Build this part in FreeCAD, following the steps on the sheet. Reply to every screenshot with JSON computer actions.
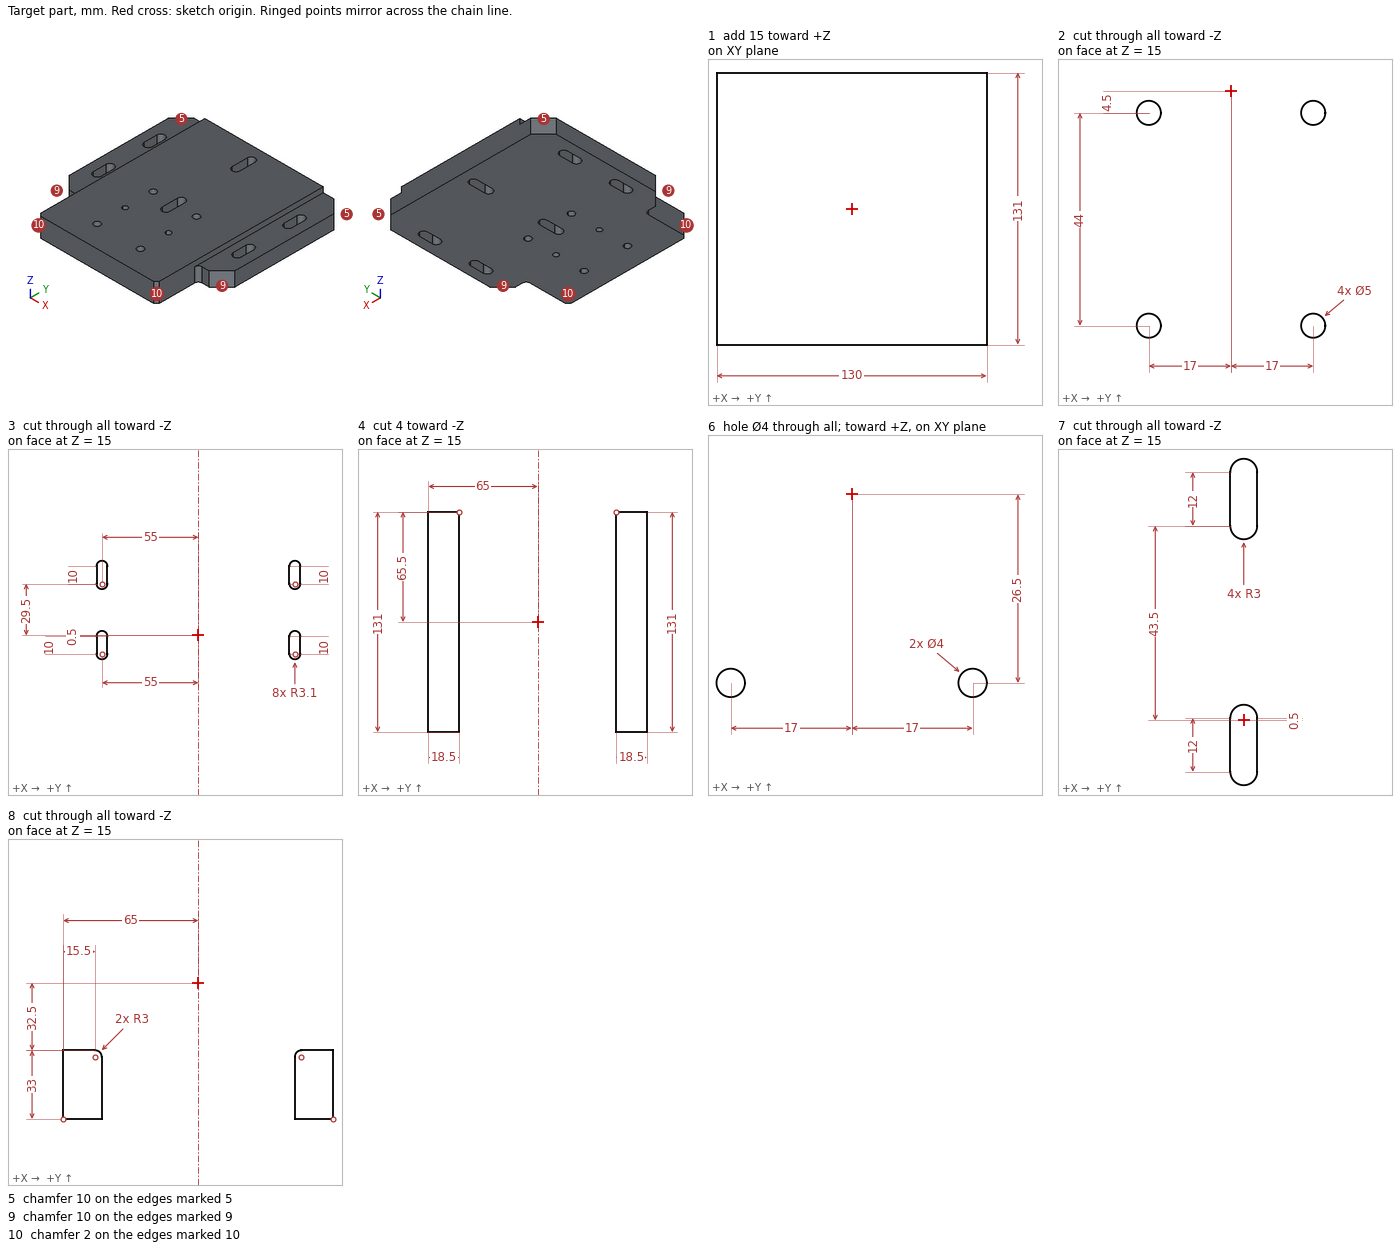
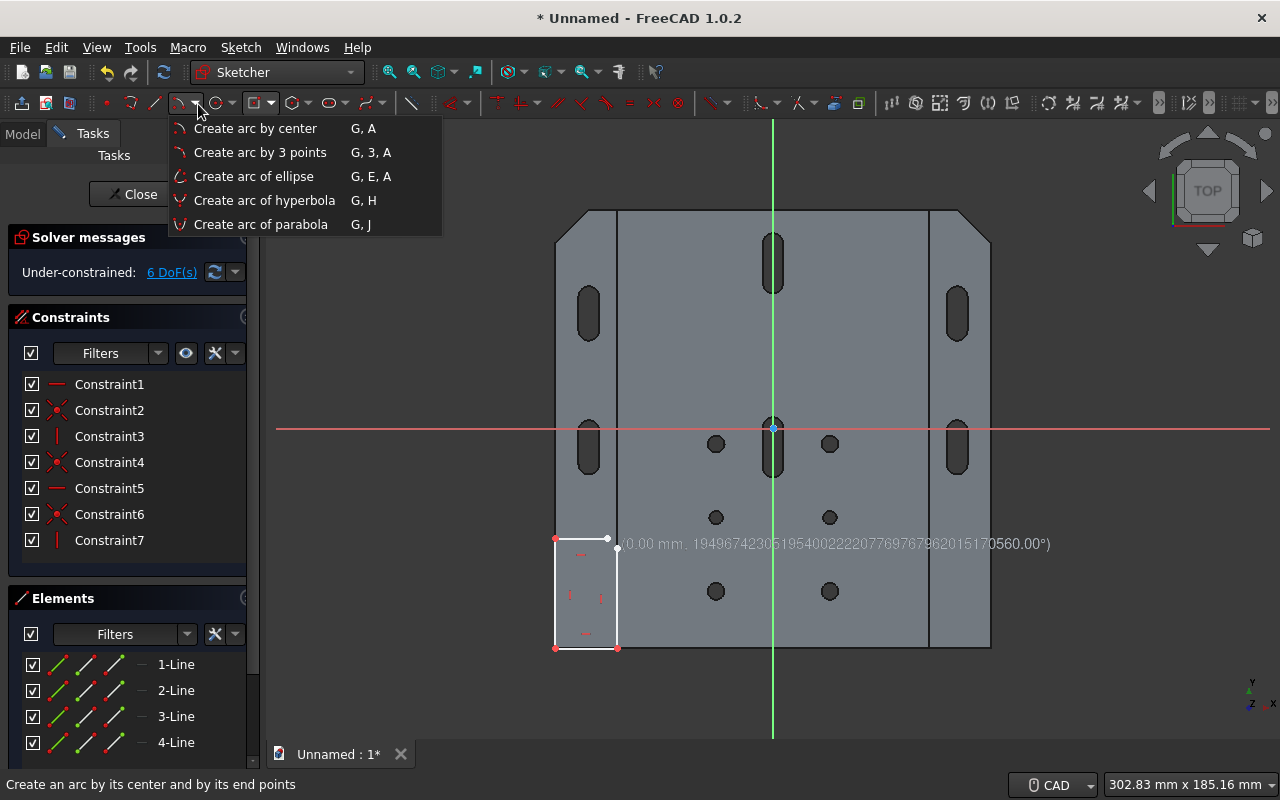
{"action": "left_click", "coordinate": [306, 152]}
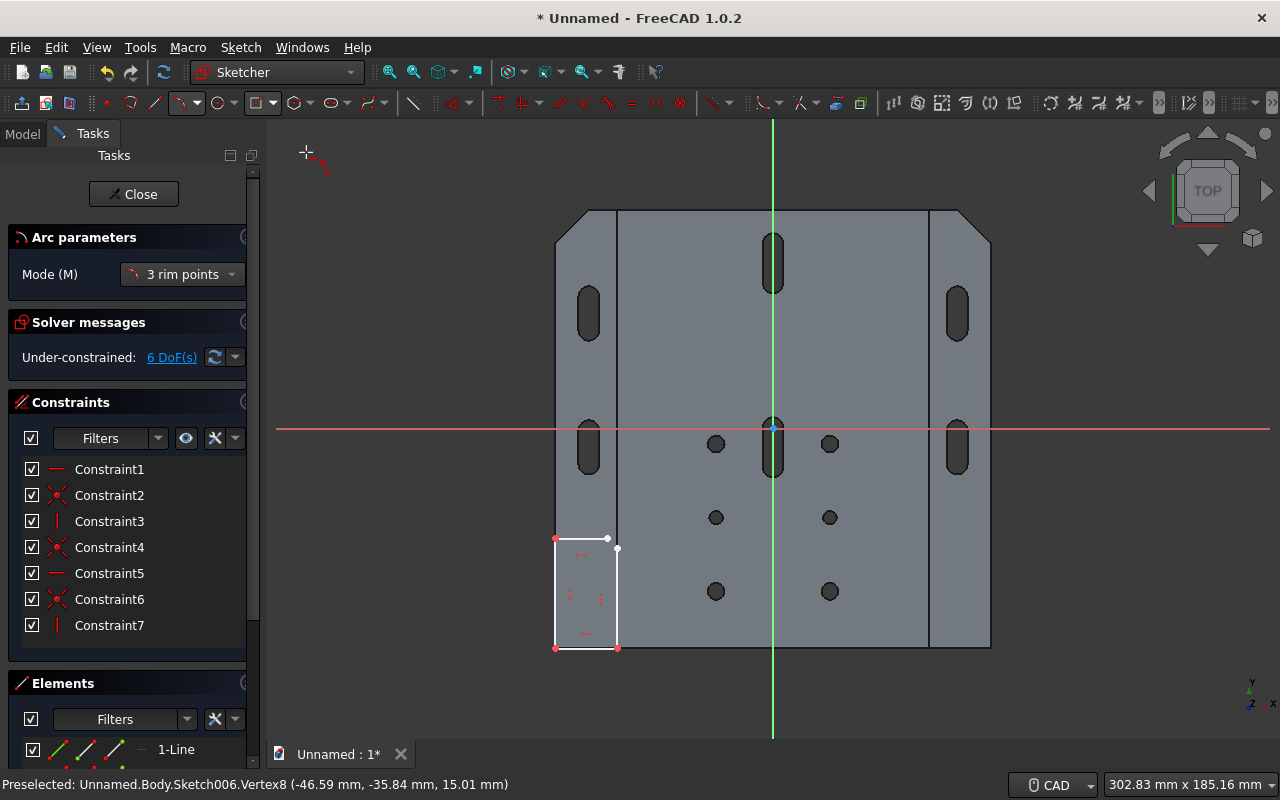
{"action": "left_click", "coordinate": [617, 549]}
{"action": "left_click", "coordinate": [607, 539]}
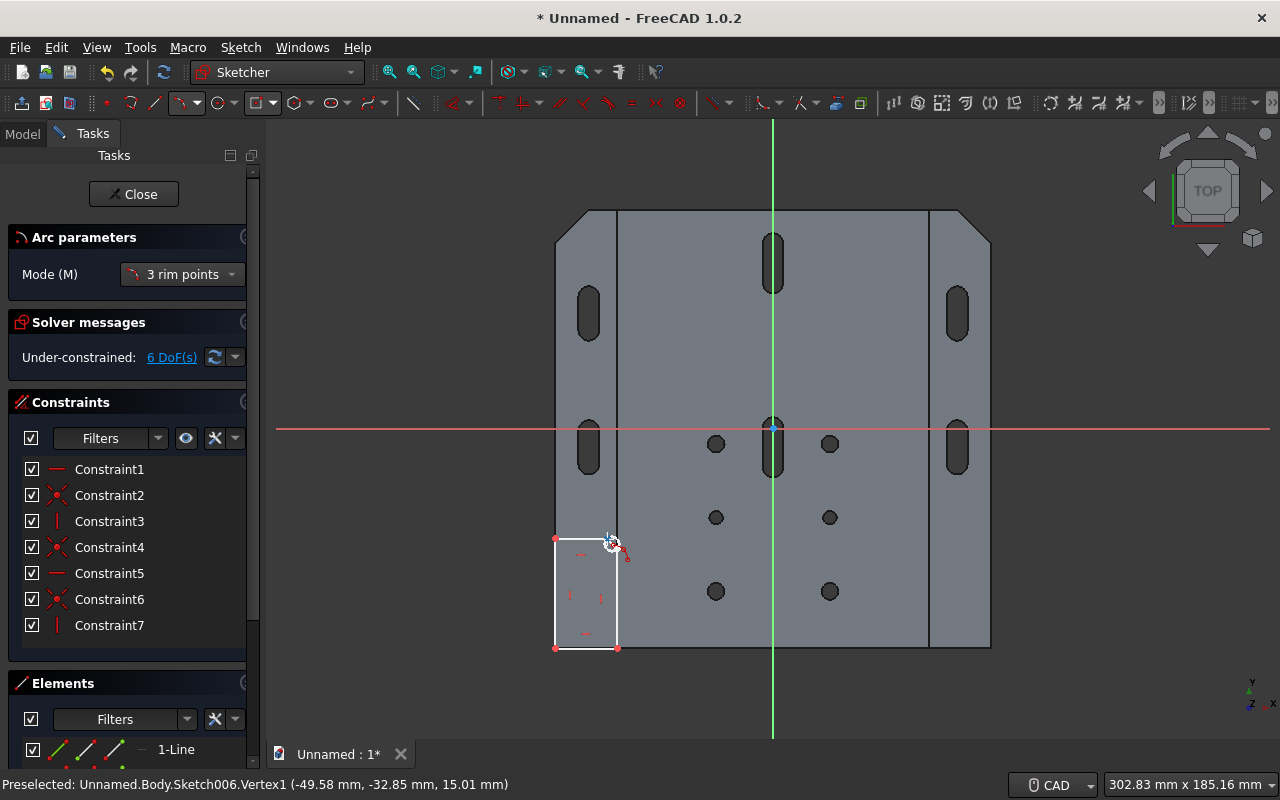
{"action": "scroll", "coordinate": [614, 541], "scroll_direction": "up", "scroll_amount": 9}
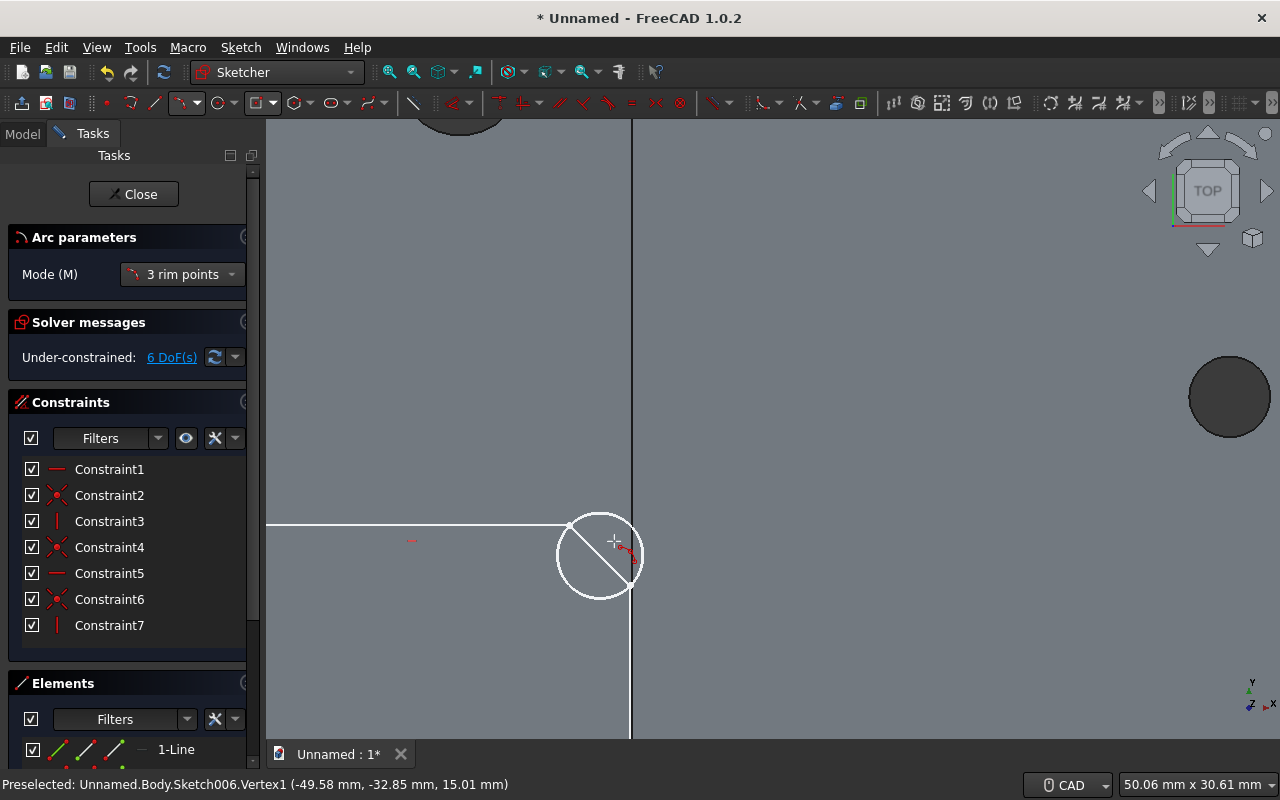
{"action": "left_click", "coordinate": [614, 536]}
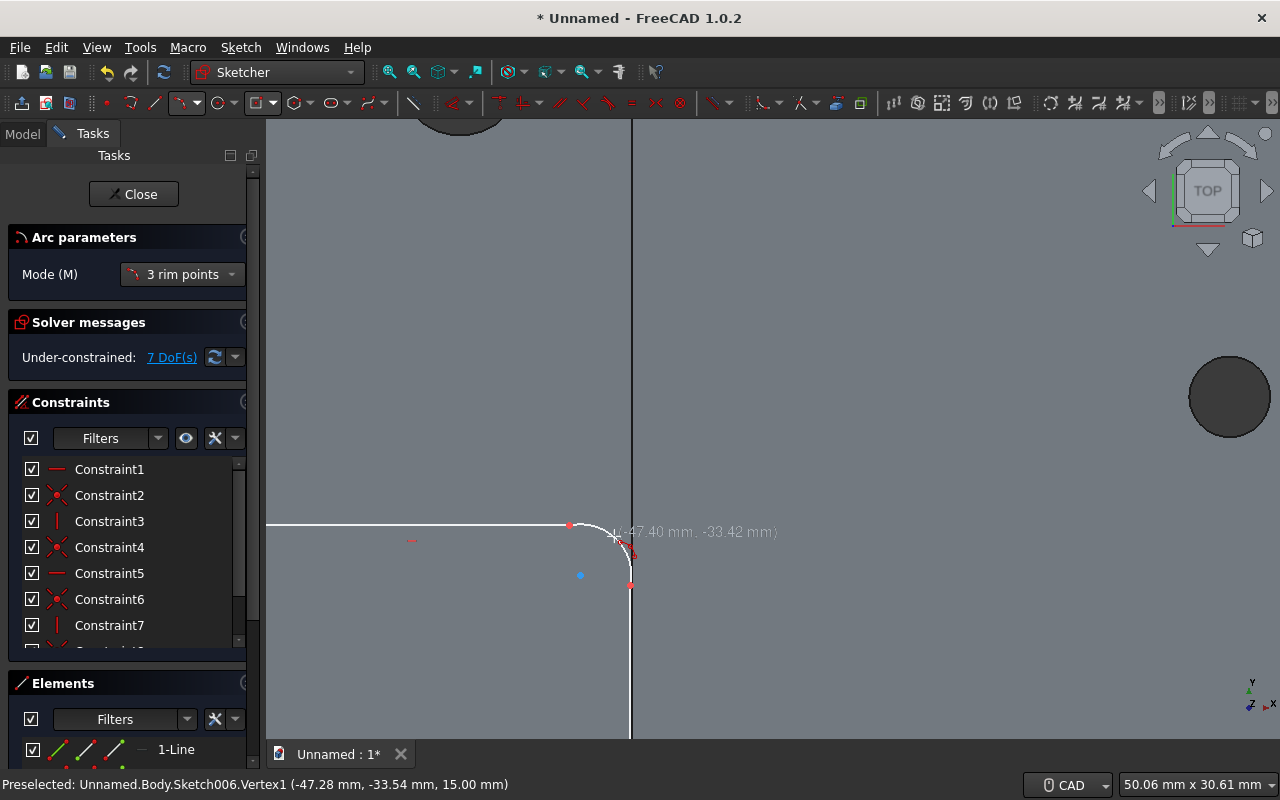
{"action": "key", "text": "g m"}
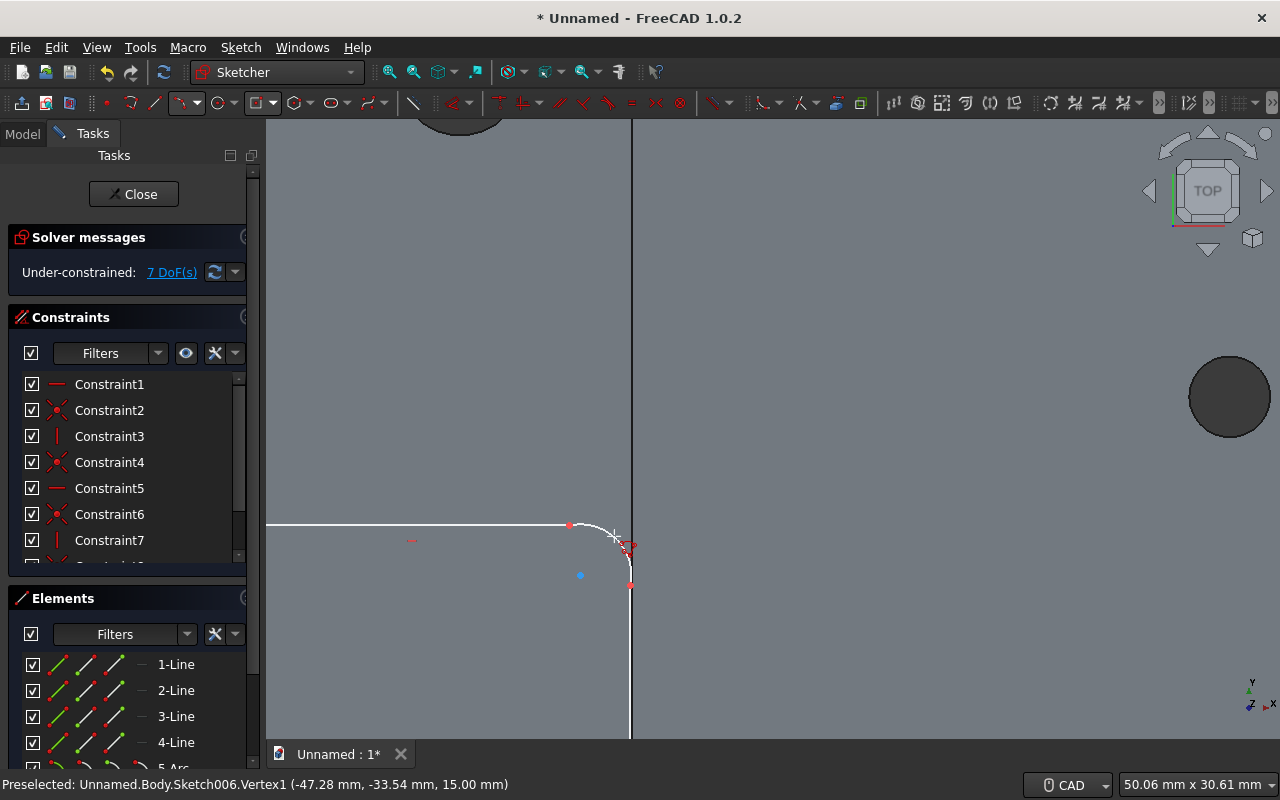
{"action": "scroll", "coordinate": [485, 405], "scroll_direction": "down", "scroll_amount": 8}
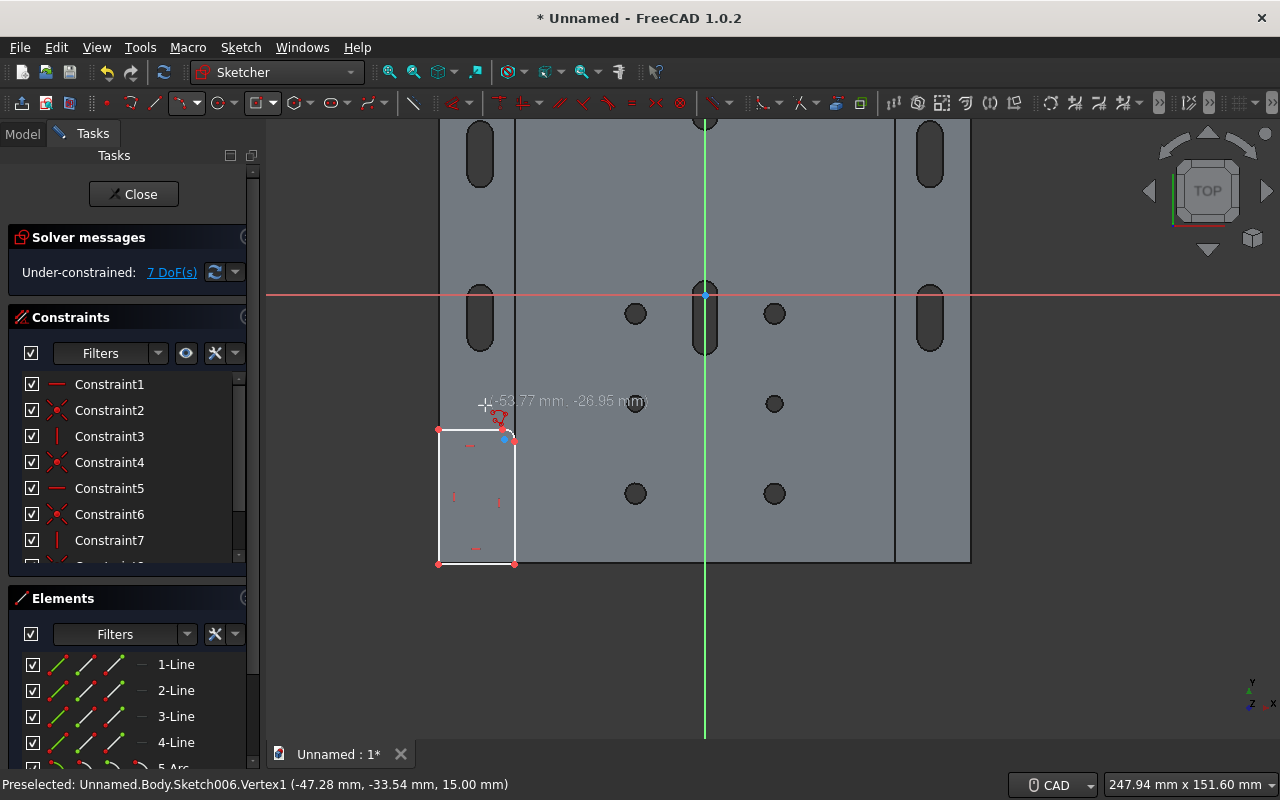
{"action": "left_click", "coordinate": [895, 441]}
{"action": "left_click", "coordinate": [895, 563]}
{"action": "left_click", "coordinate": [971, 563]}
{"action": "left_click", "coordinate": [971, 428]}
{"action": "left_click", "coordinate": [908, 428]}
{"action": "right_click", "coordinate": [908, 428]}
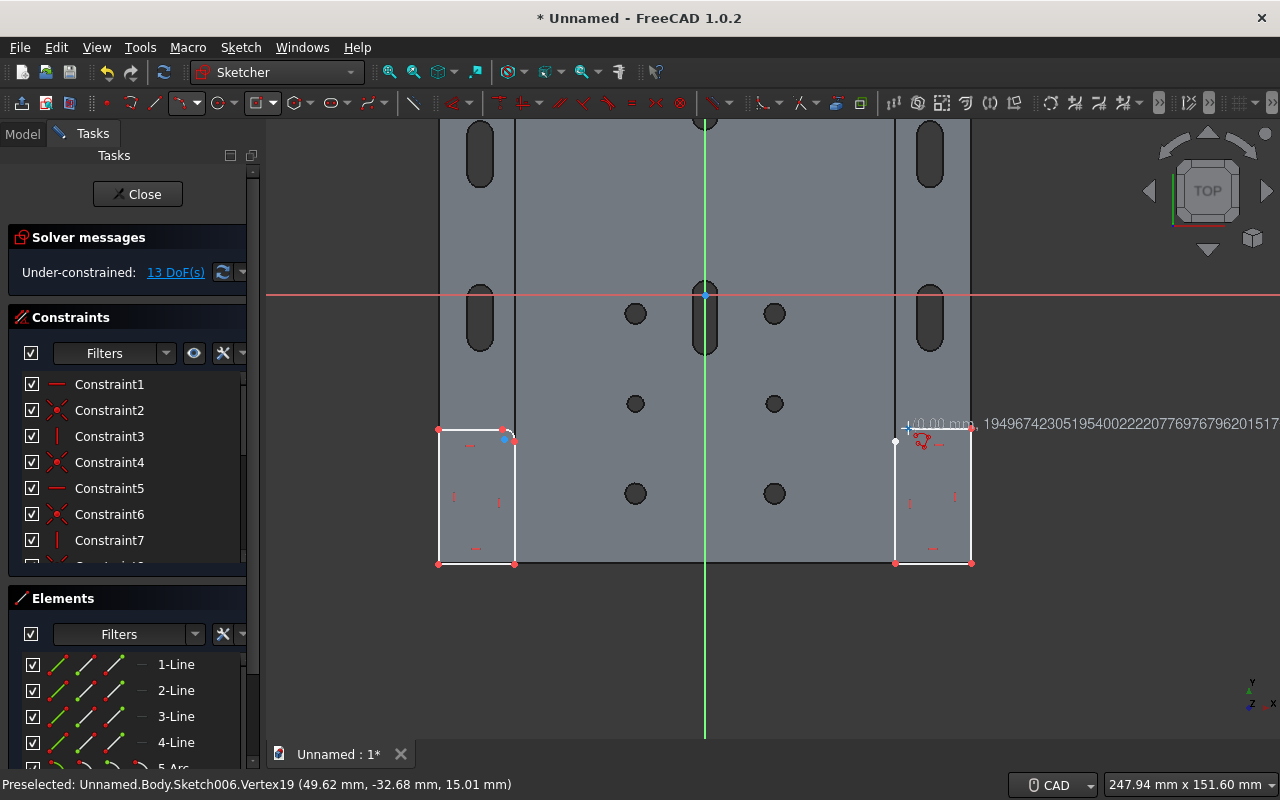
{"action": "left_click", "coordinate": [180, 104]}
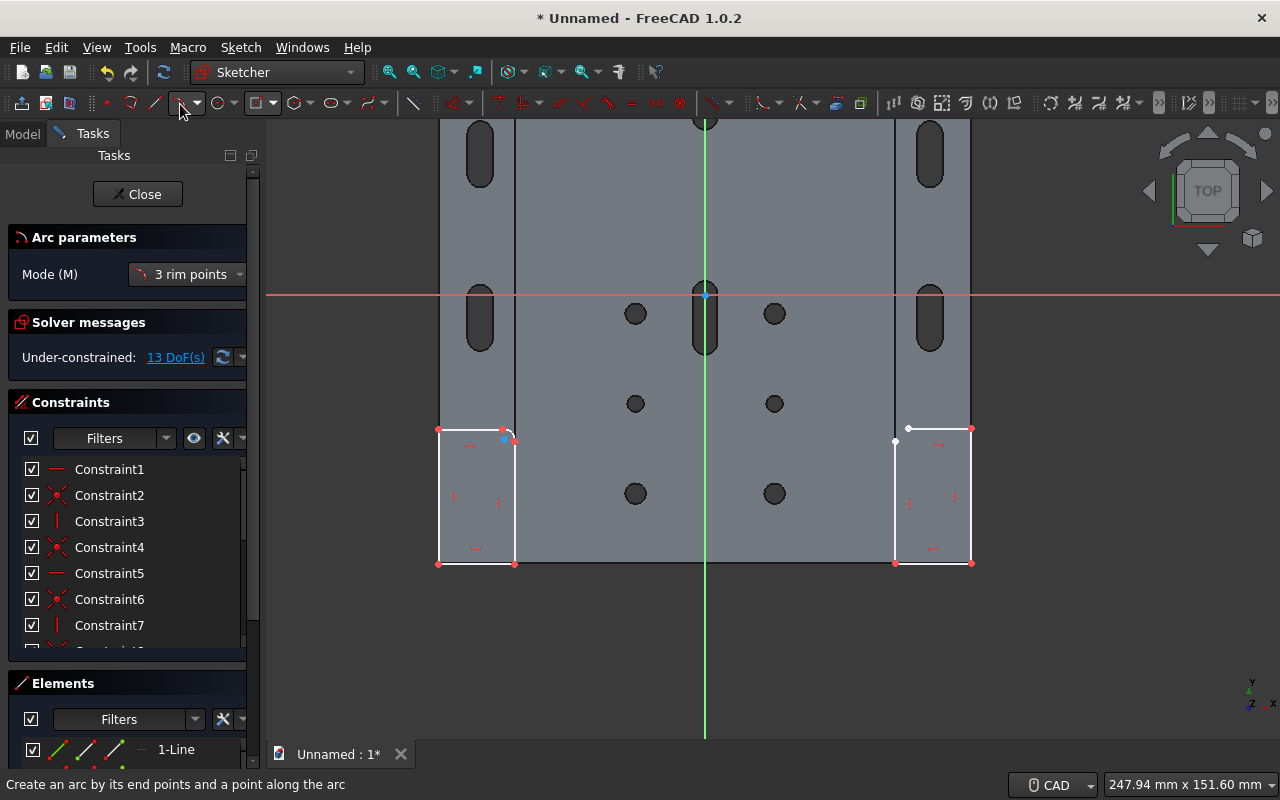
{"action": "left_click", "coordinate": [908, 429]}
{"action": "left_click", "coordinate": [895, 442]}